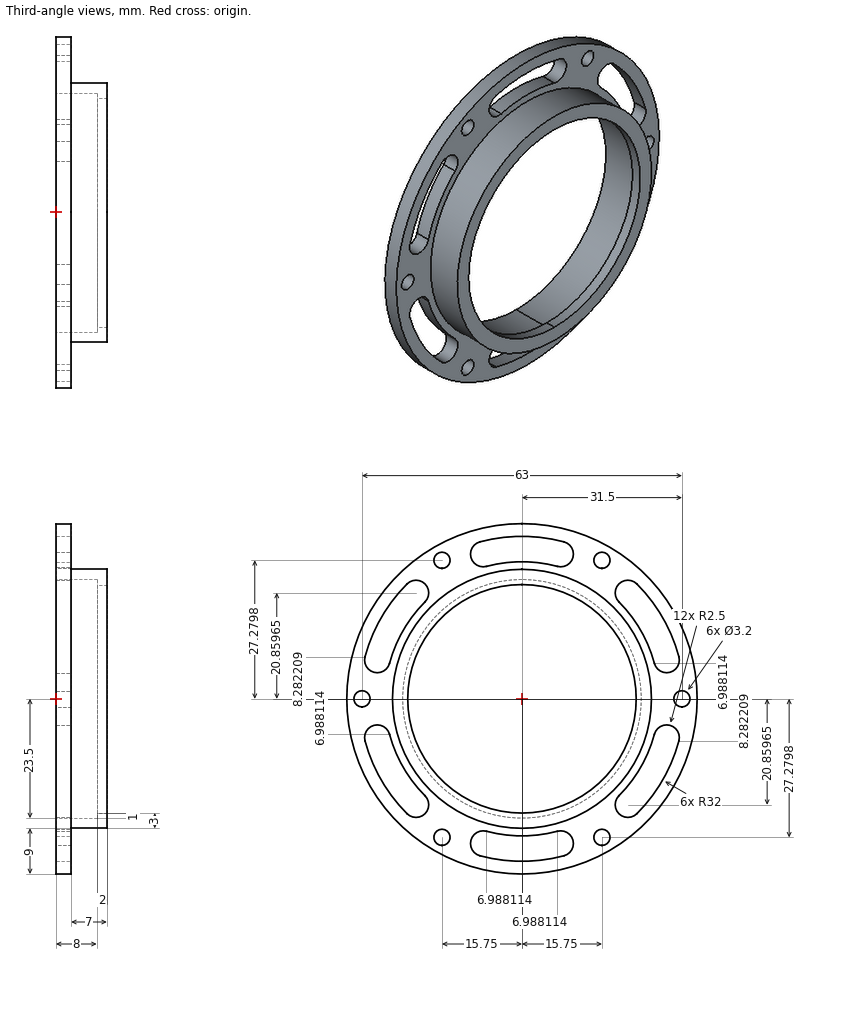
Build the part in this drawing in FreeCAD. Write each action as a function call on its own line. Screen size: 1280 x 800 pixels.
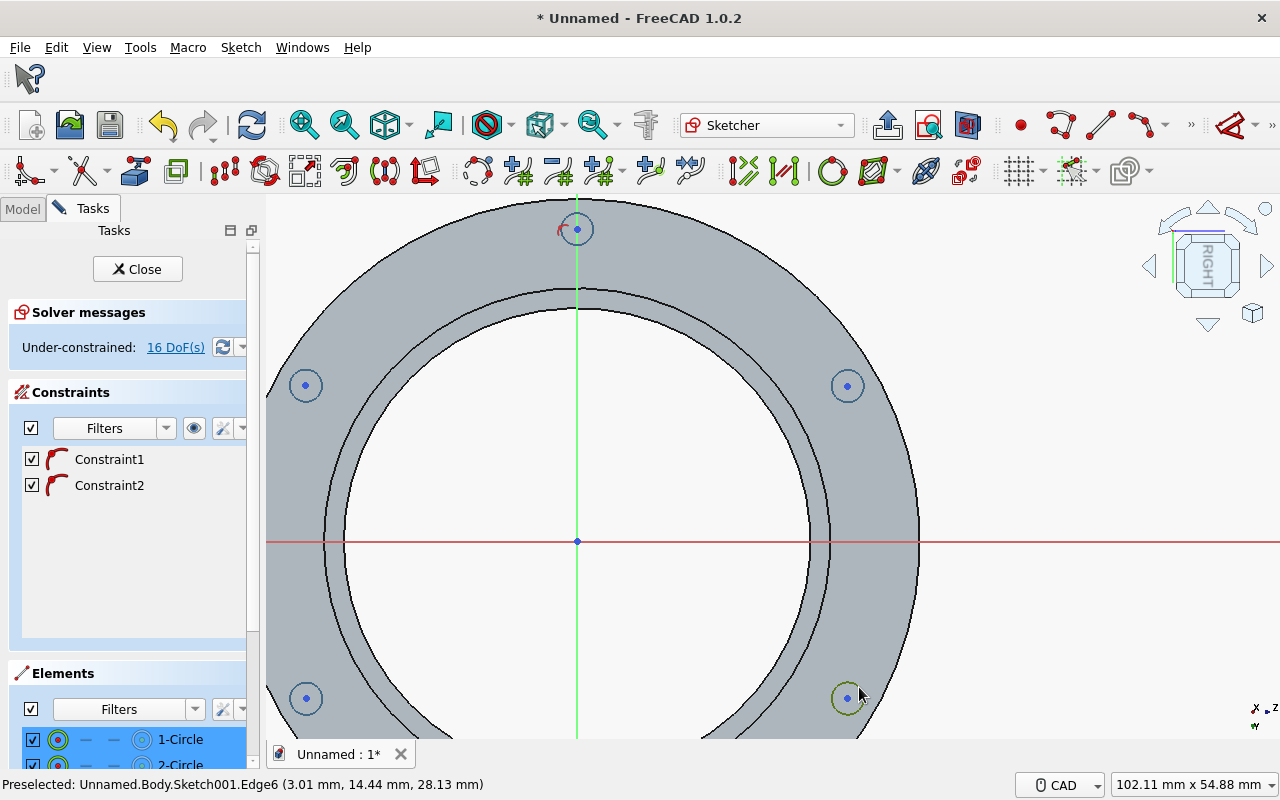
key(e)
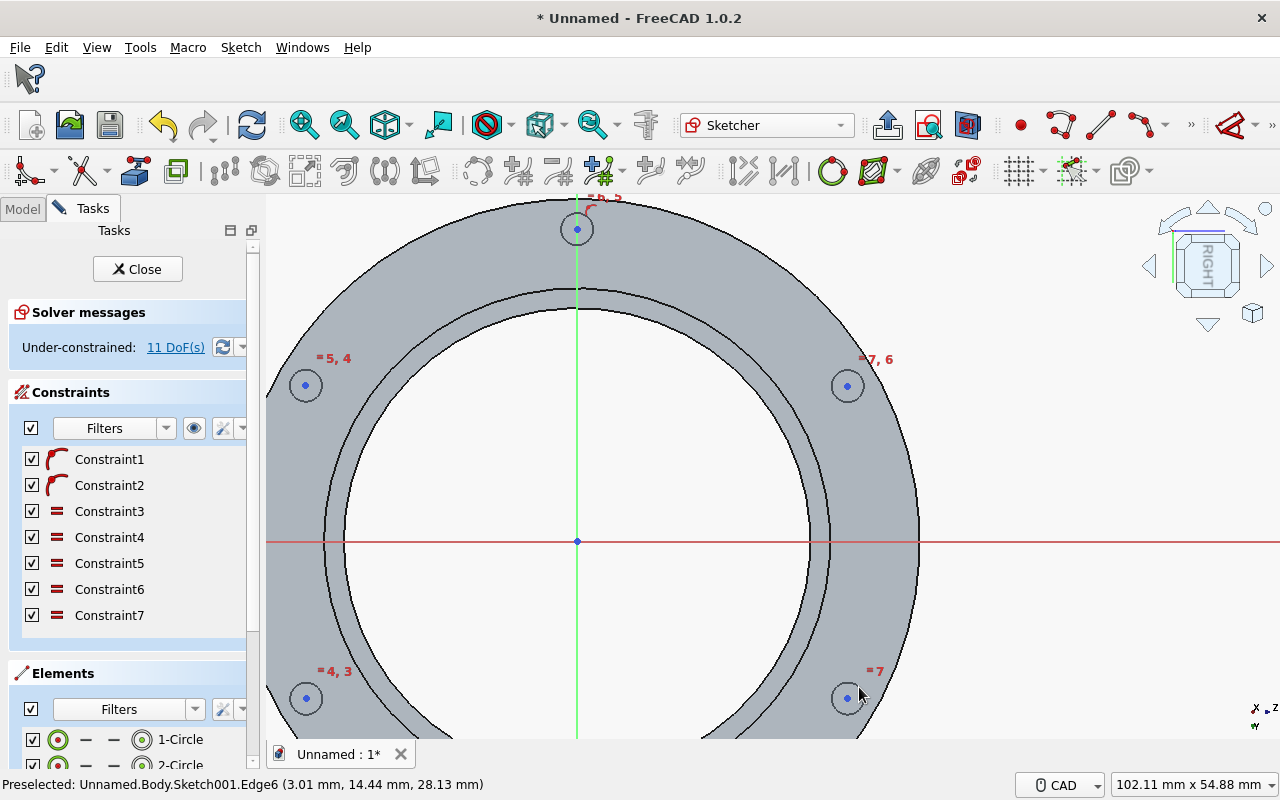
click(306, 699)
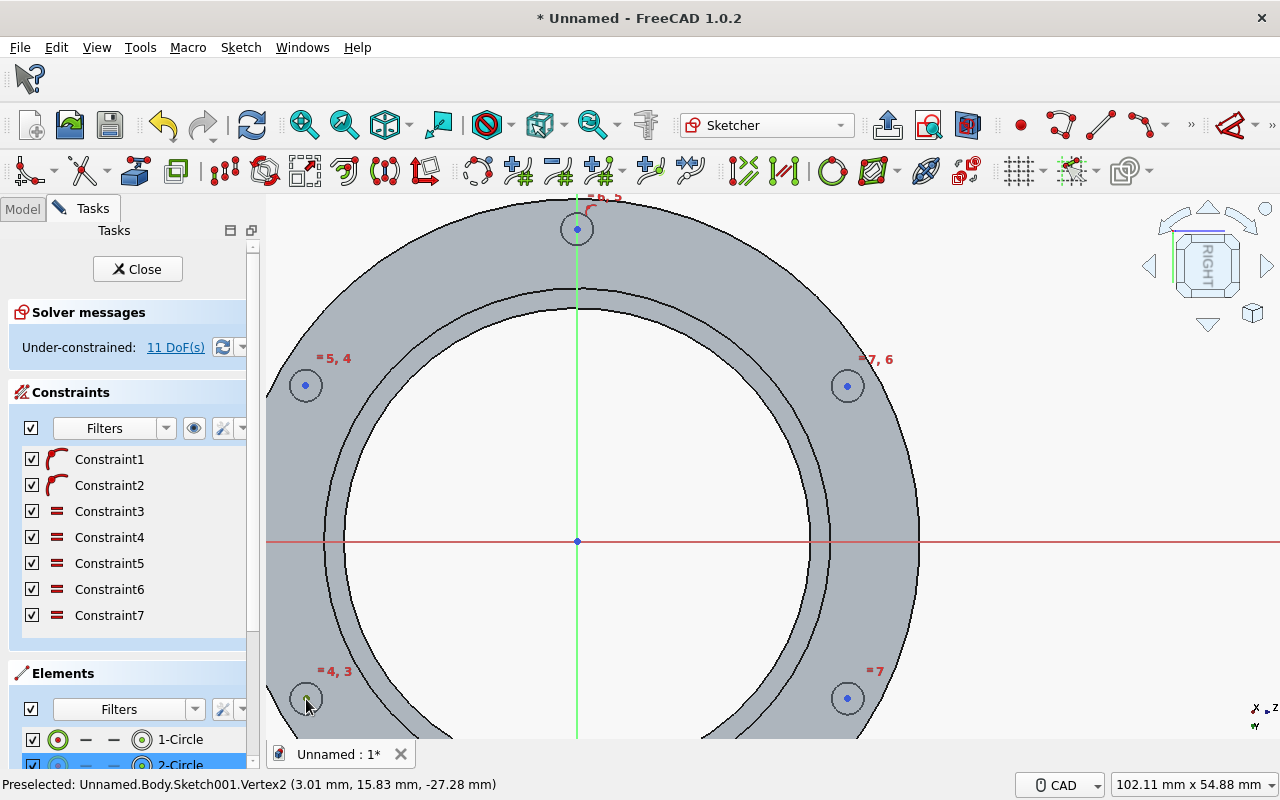
click(306, 386)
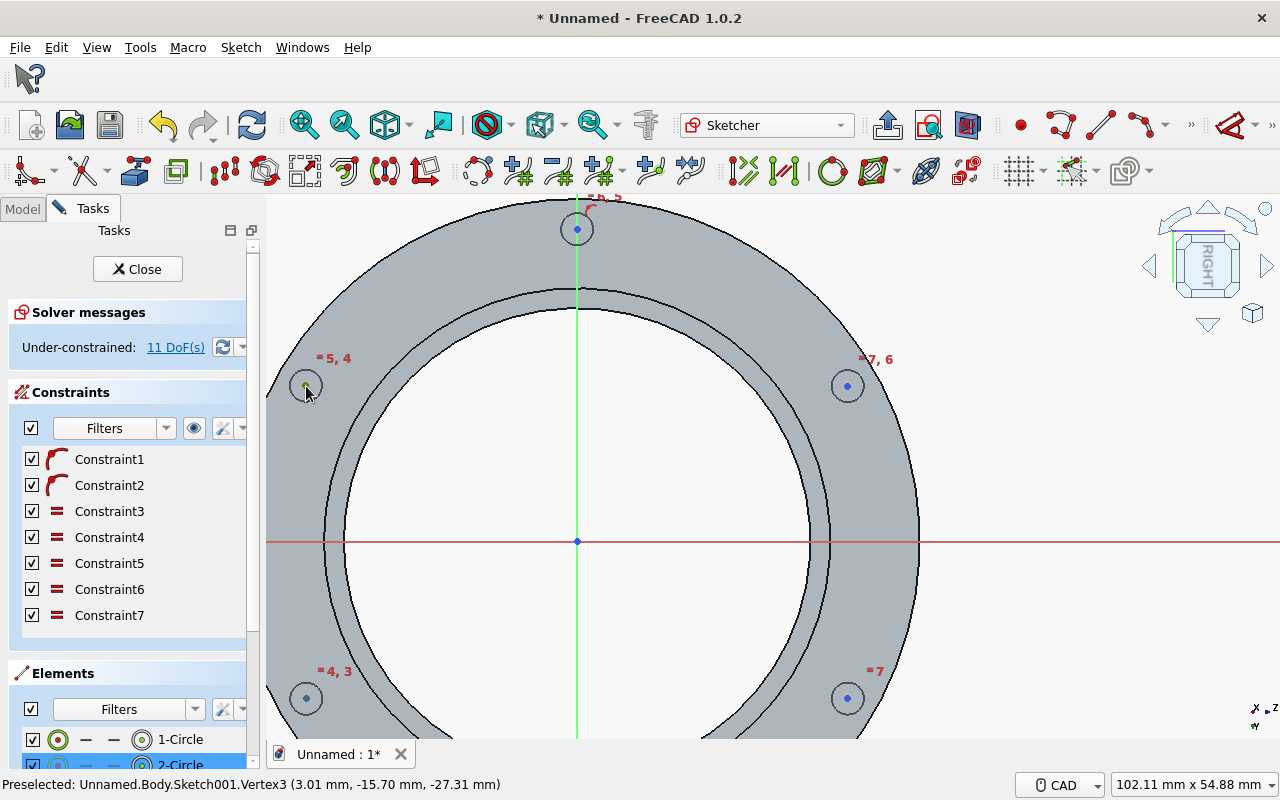
key(v)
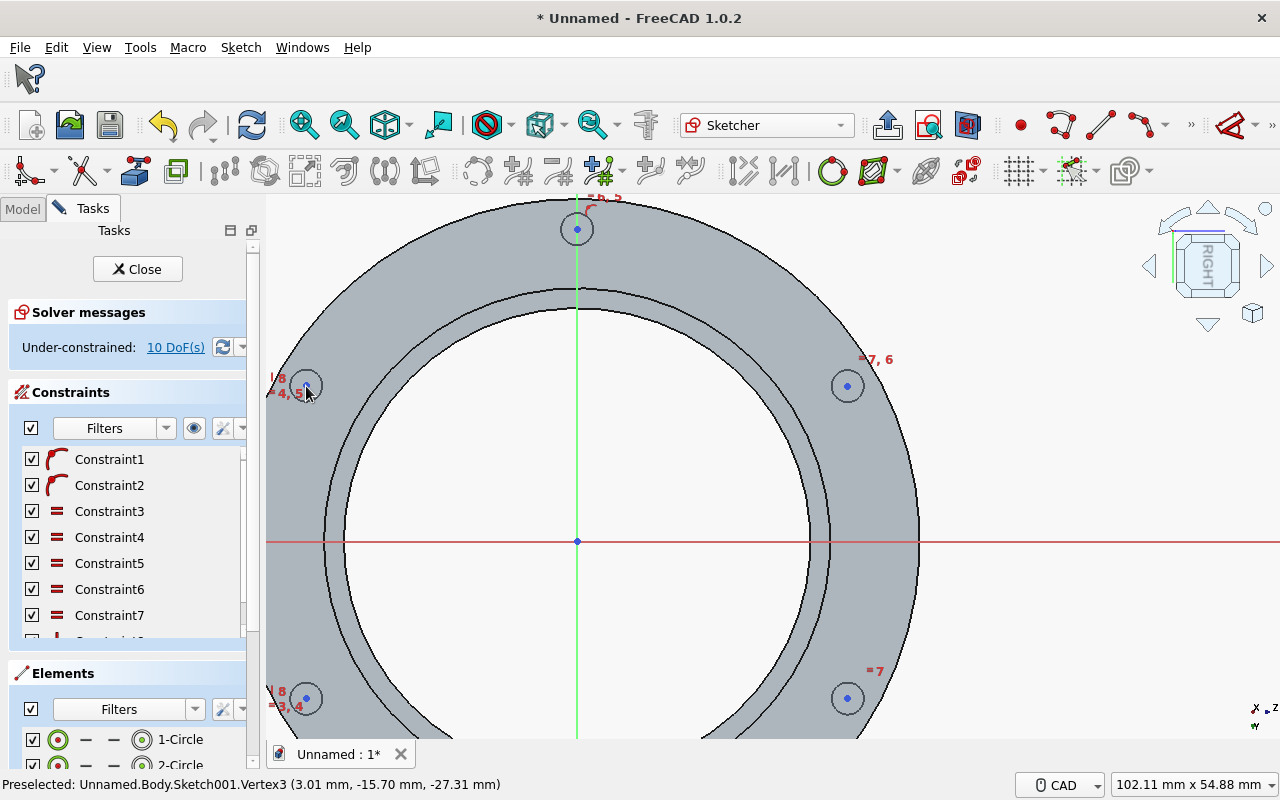
click(306, 386)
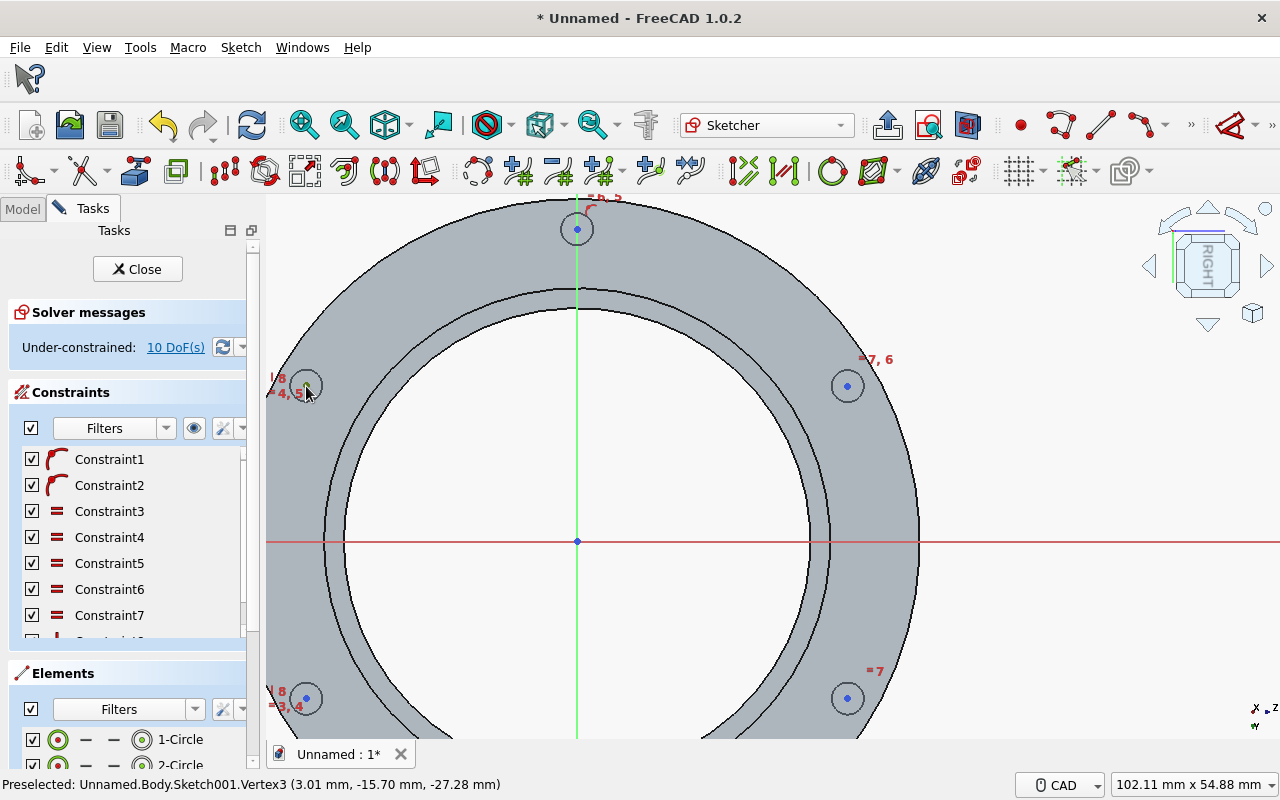
click(848, 386)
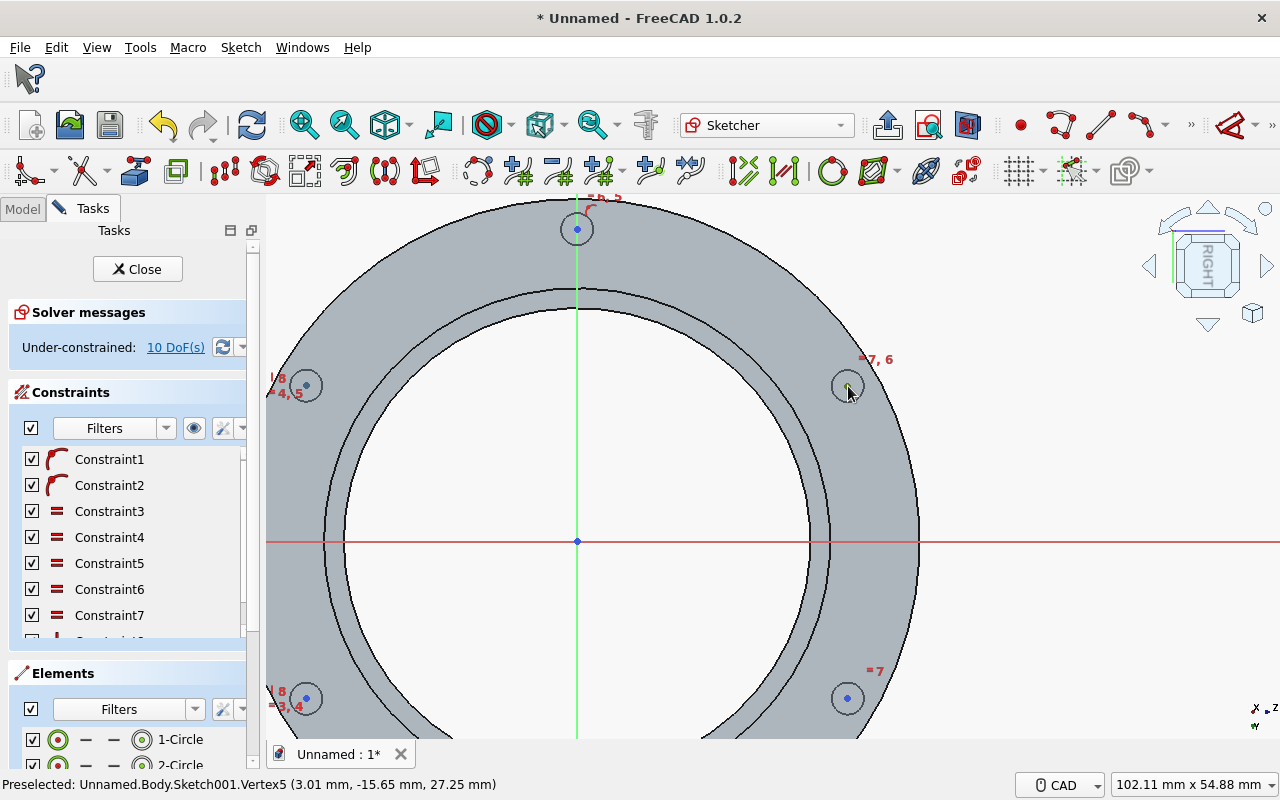
key(h)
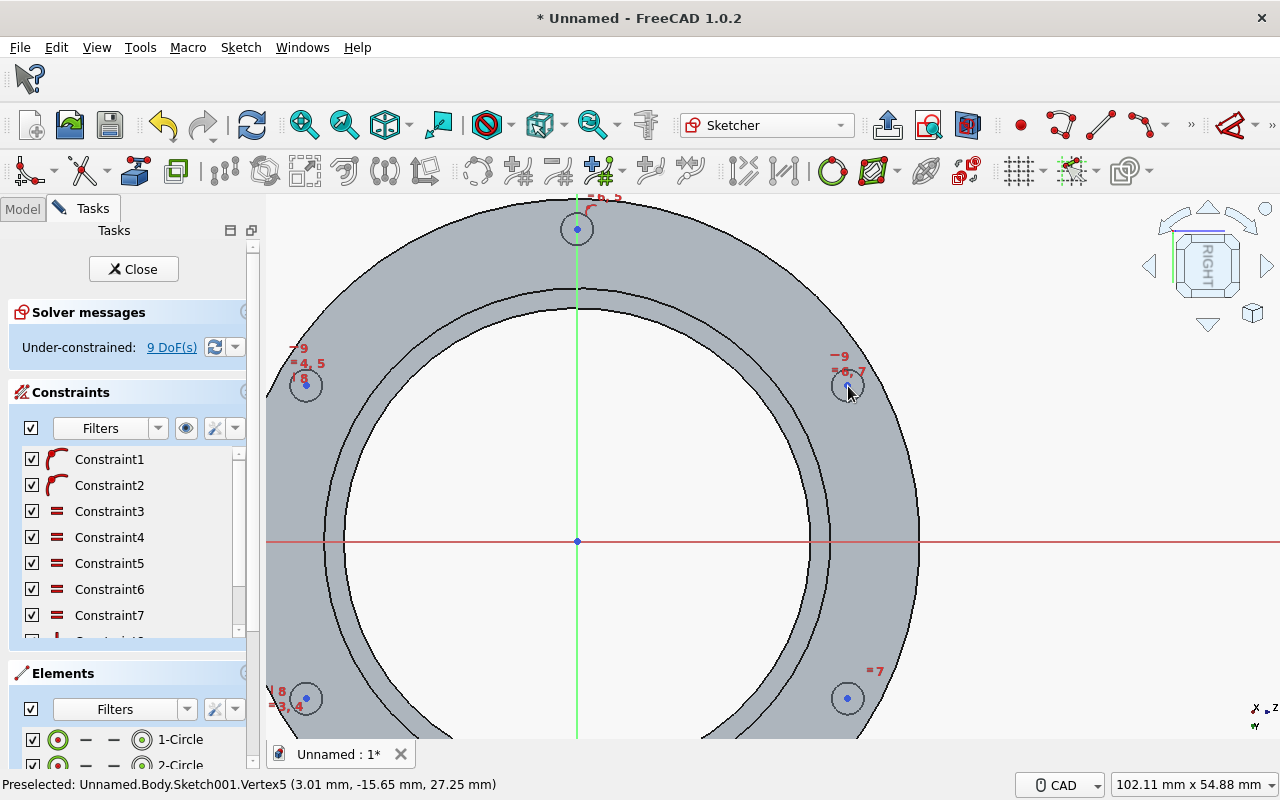
click(848, 386)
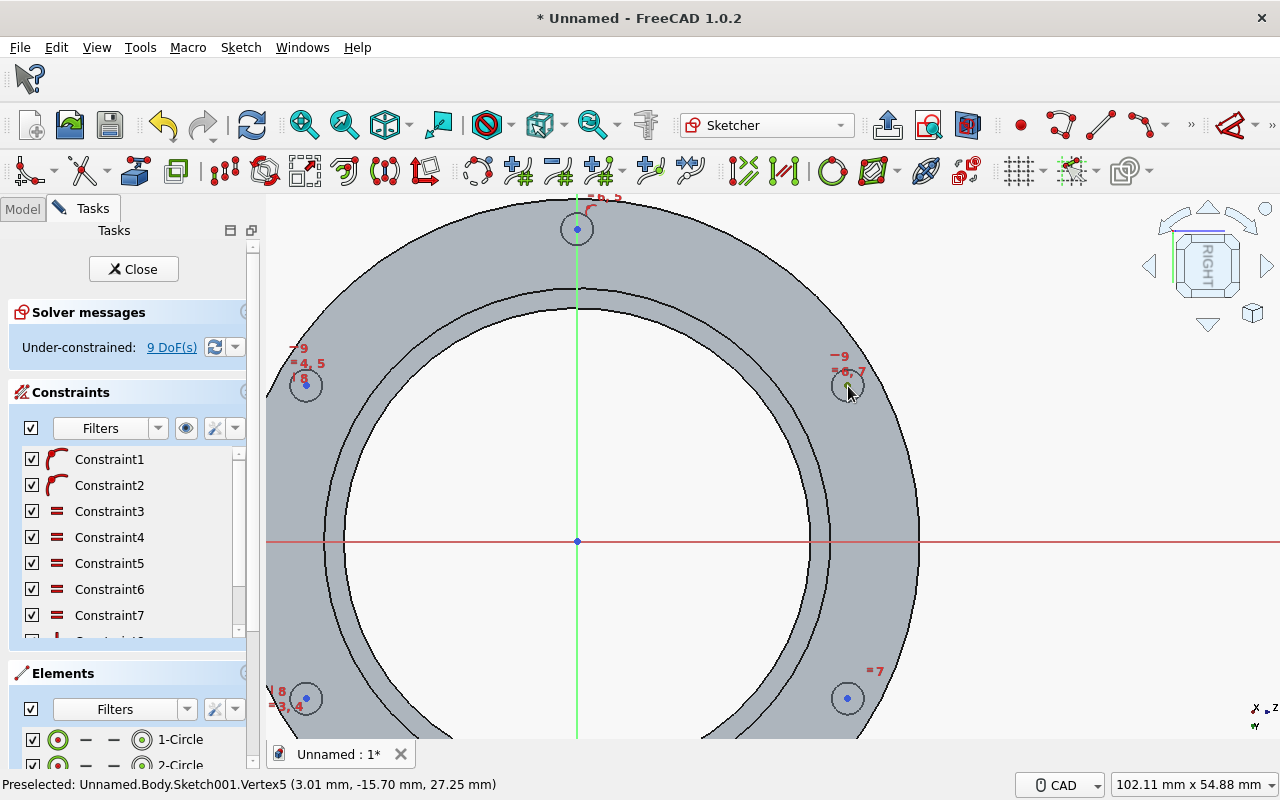
click(848, 699)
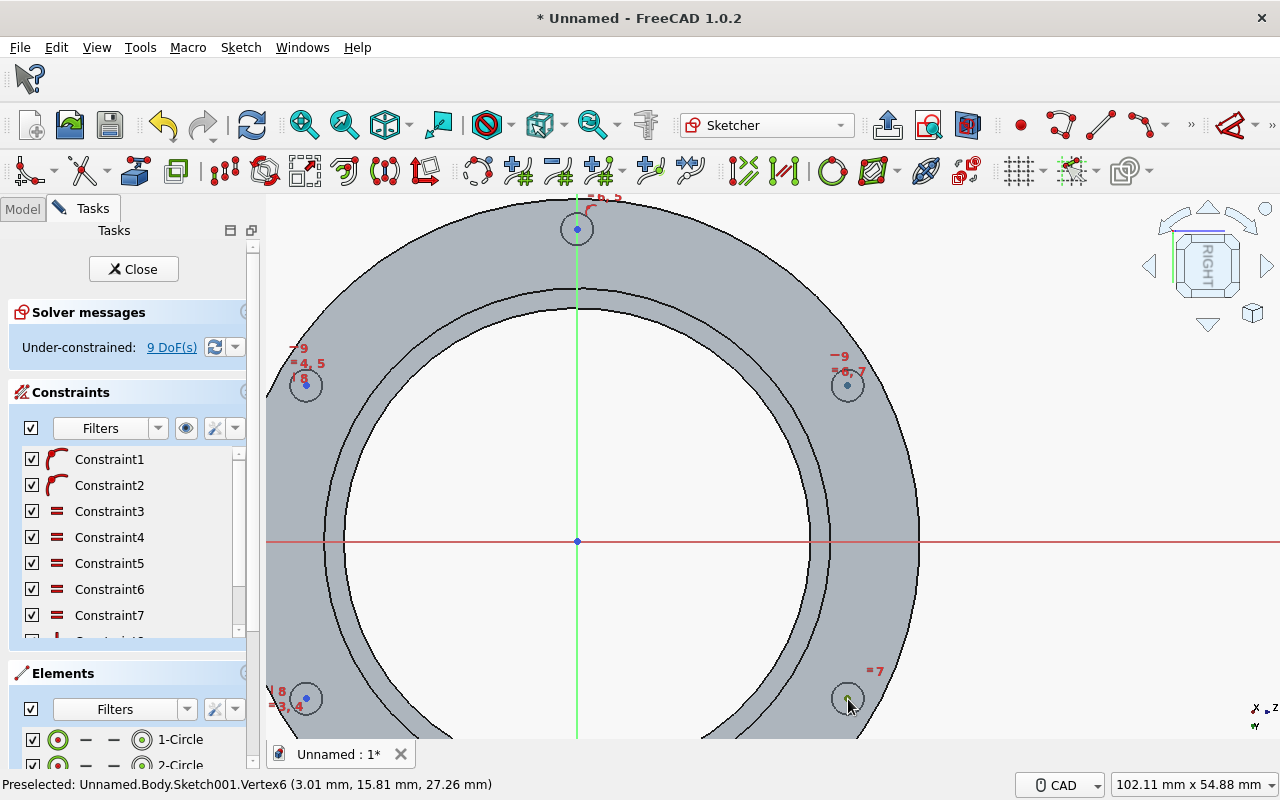
key(v)